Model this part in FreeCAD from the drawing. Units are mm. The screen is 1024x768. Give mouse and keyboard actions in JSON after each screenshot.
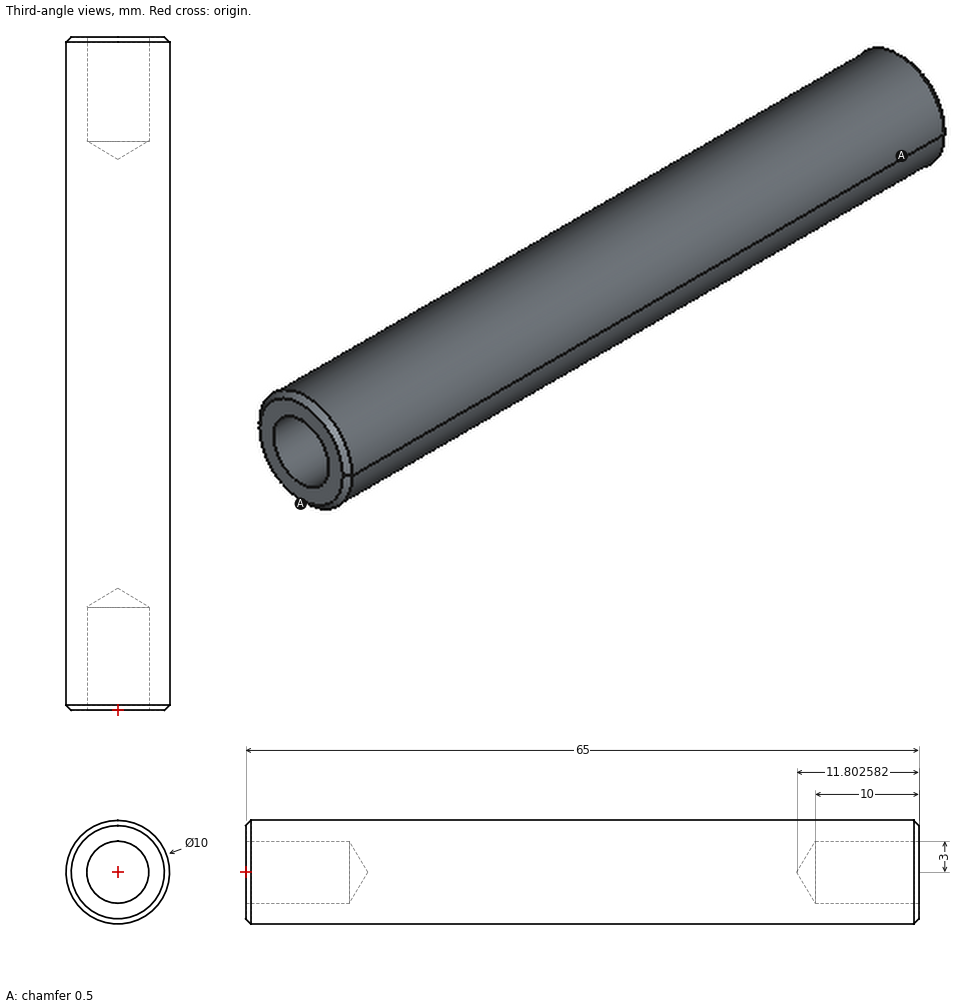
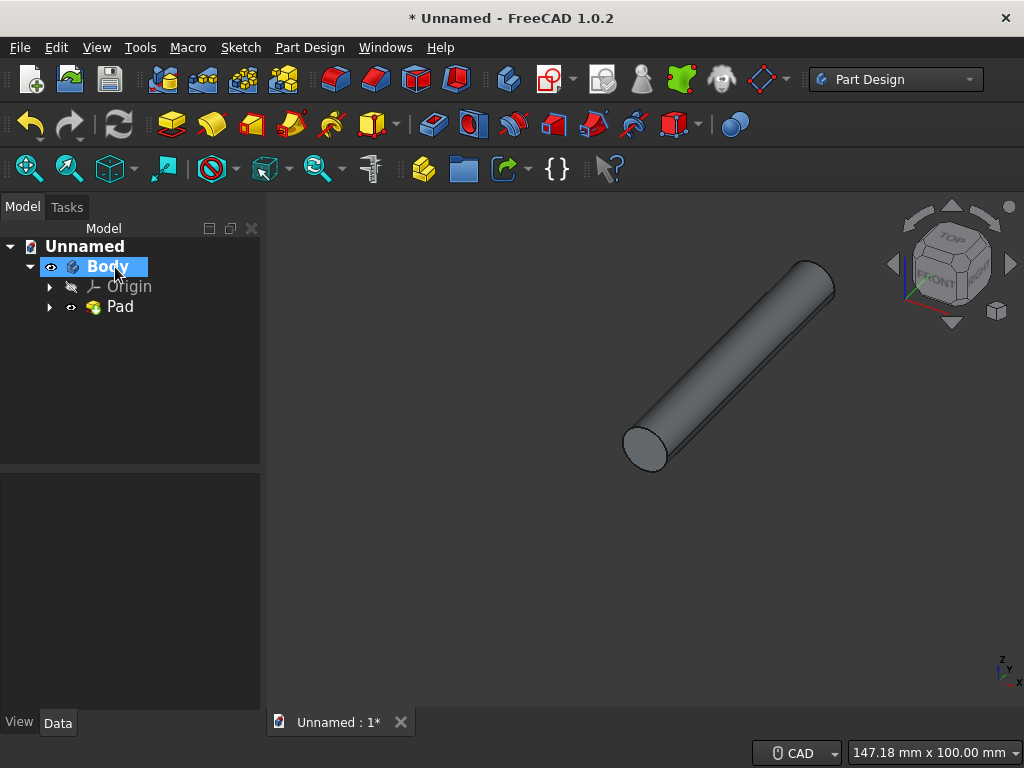
{"action": "left_click", "coordinate": [30, 170]}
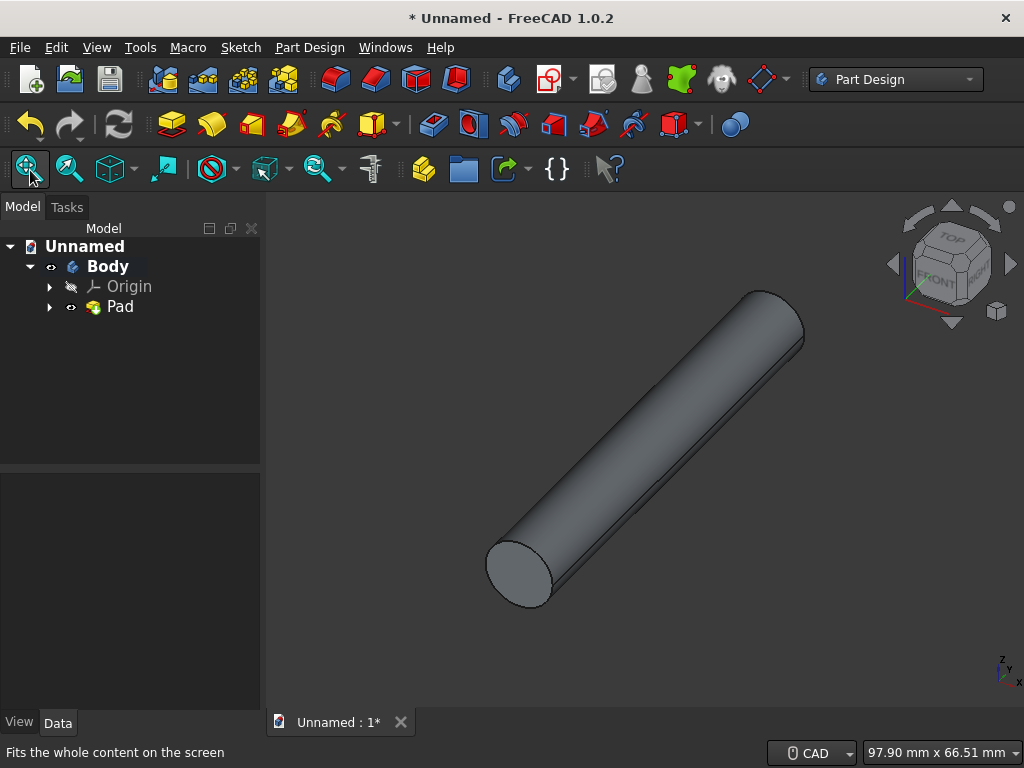
{"action": "left_click", "coordinate": [550, 80]}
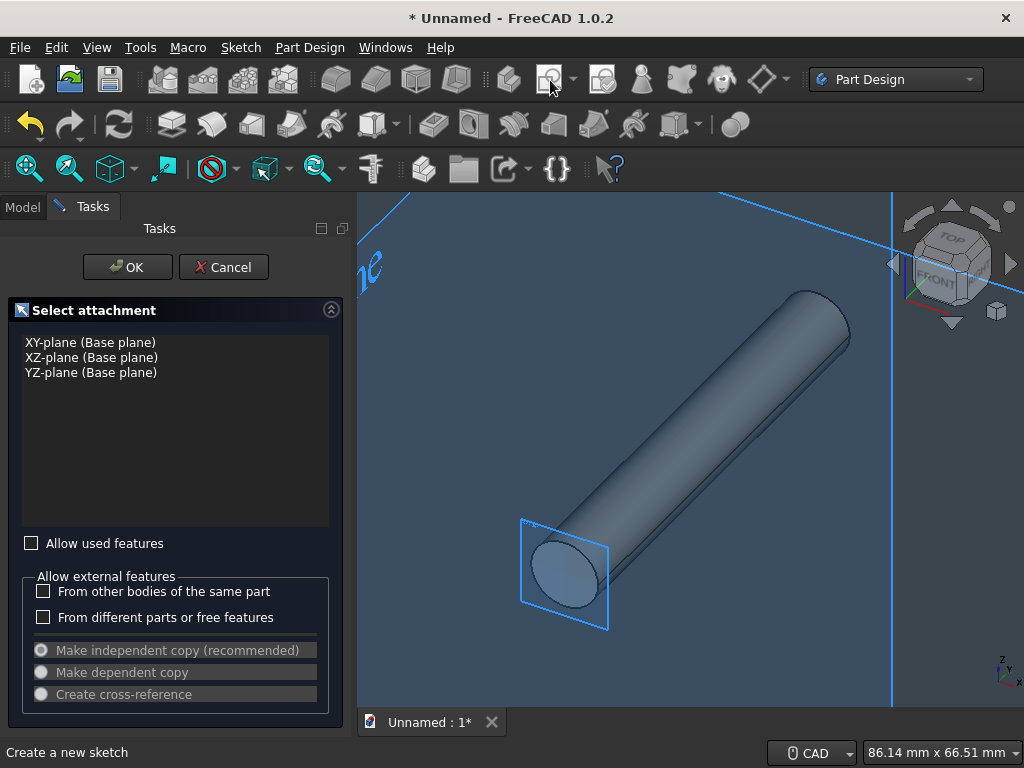
{"action": "left_click", "coordinate": [82, 372]}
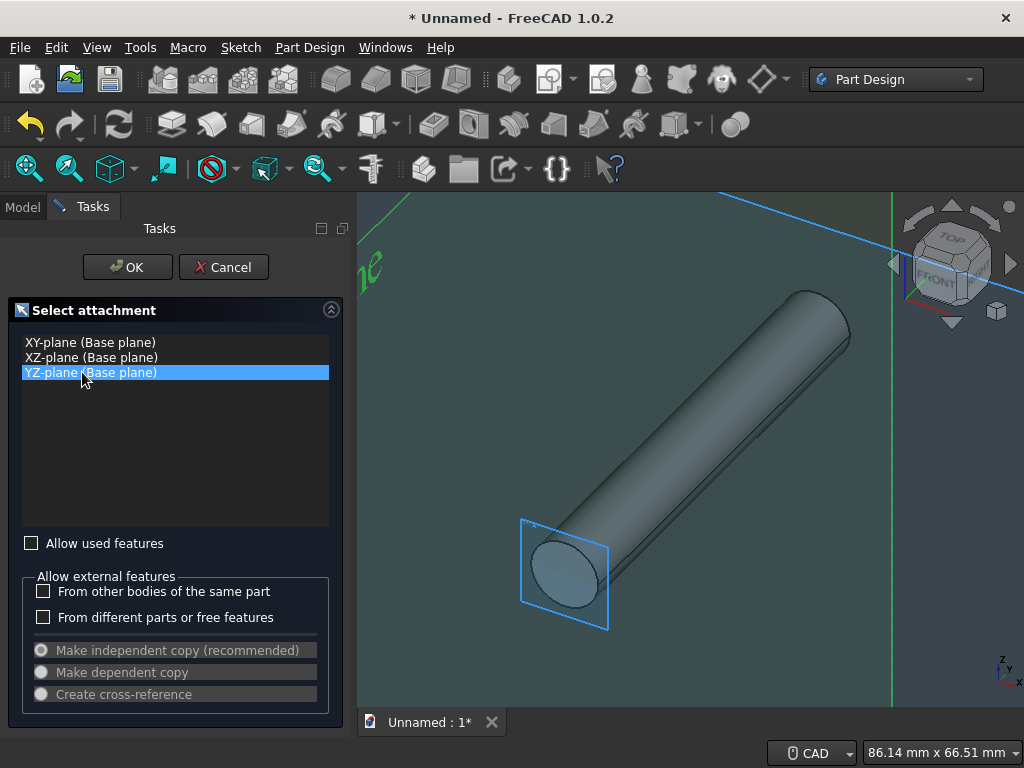
{"action": "left_click", "coordinate": [128, 267]}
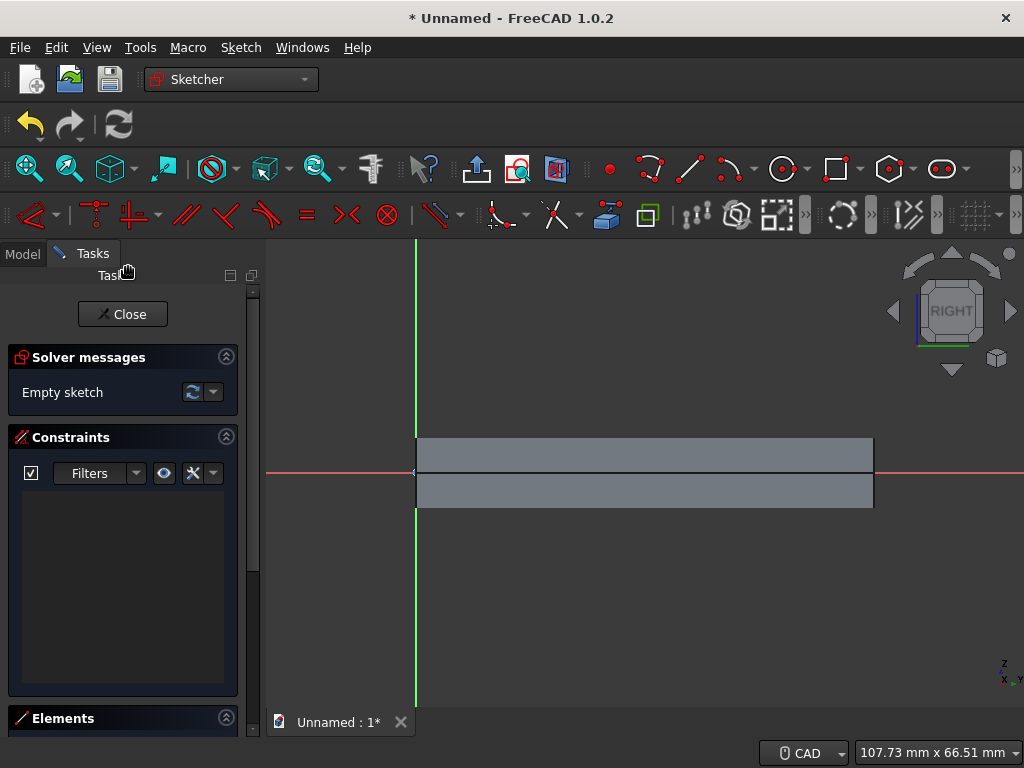
{"action": "left_click", "coordinate": [558, 170]}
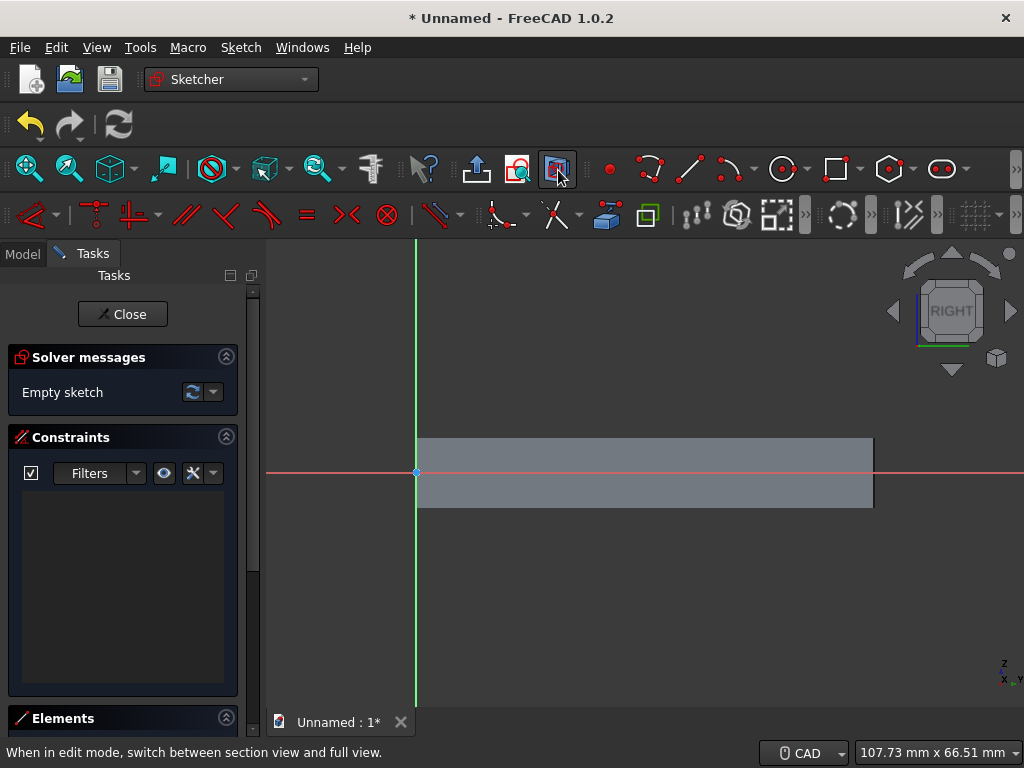
{"action": "scroll", "coordinate": [576, 473], "scroll_direction": "down", "scroll_amount": 5}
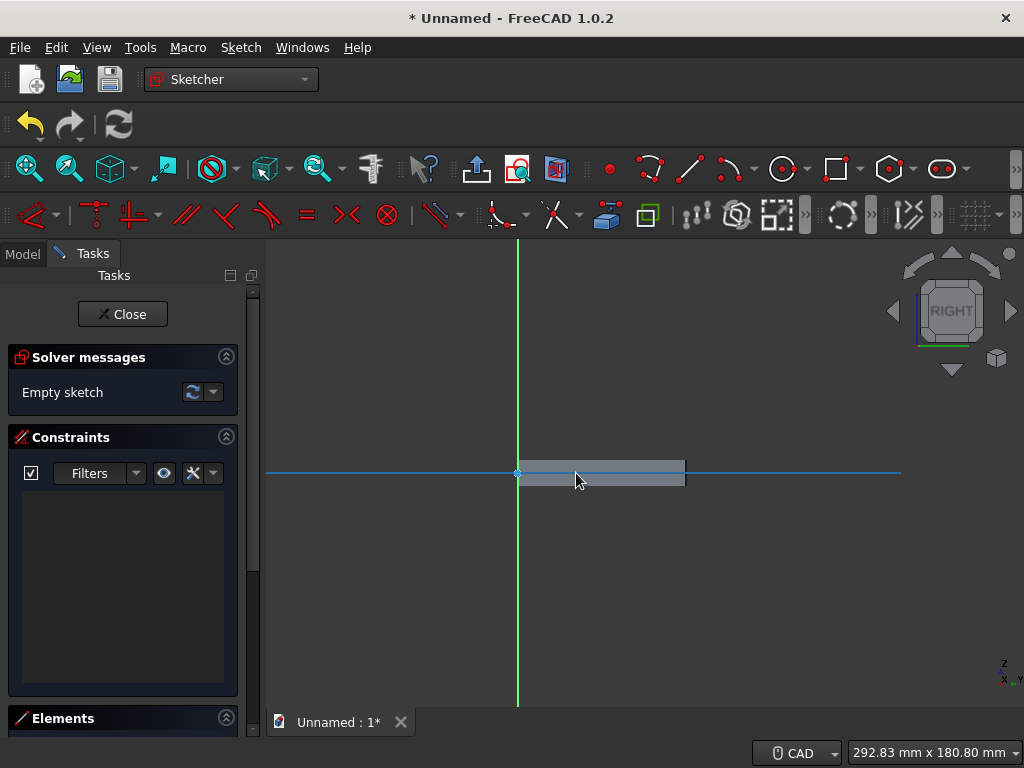
{"action": "scroll", "coordinate": [678, 469], "scroll_direction": "up", "scroll_amount": 13}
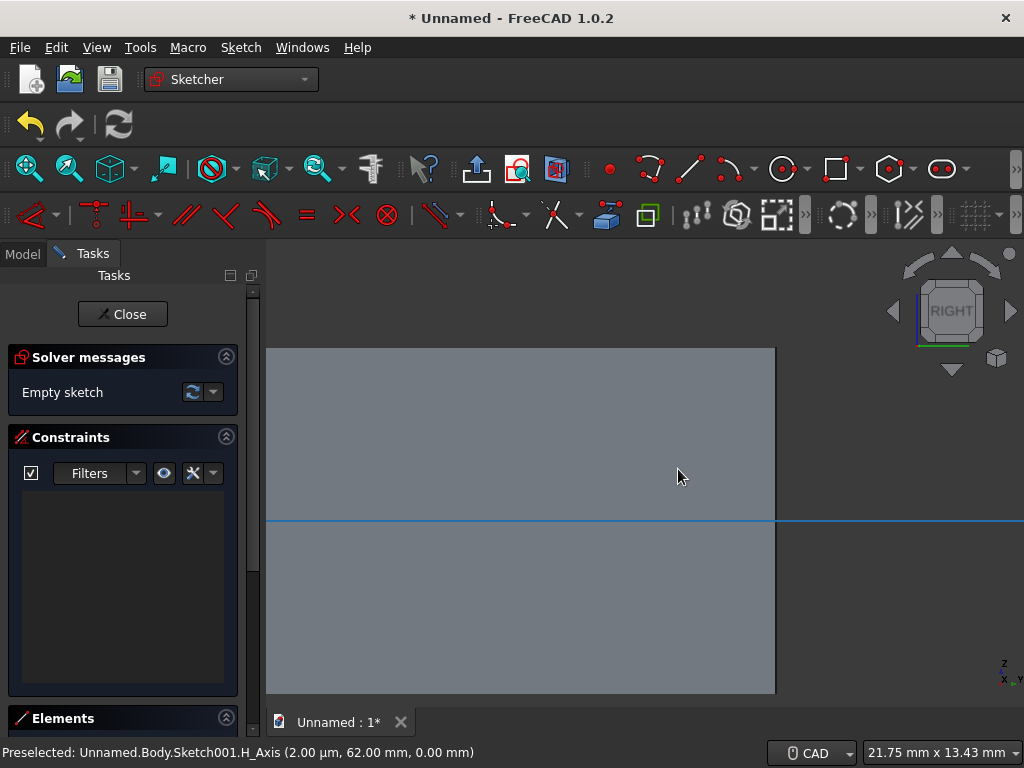
{"action": "left_click", "coordinate": [650, 170]}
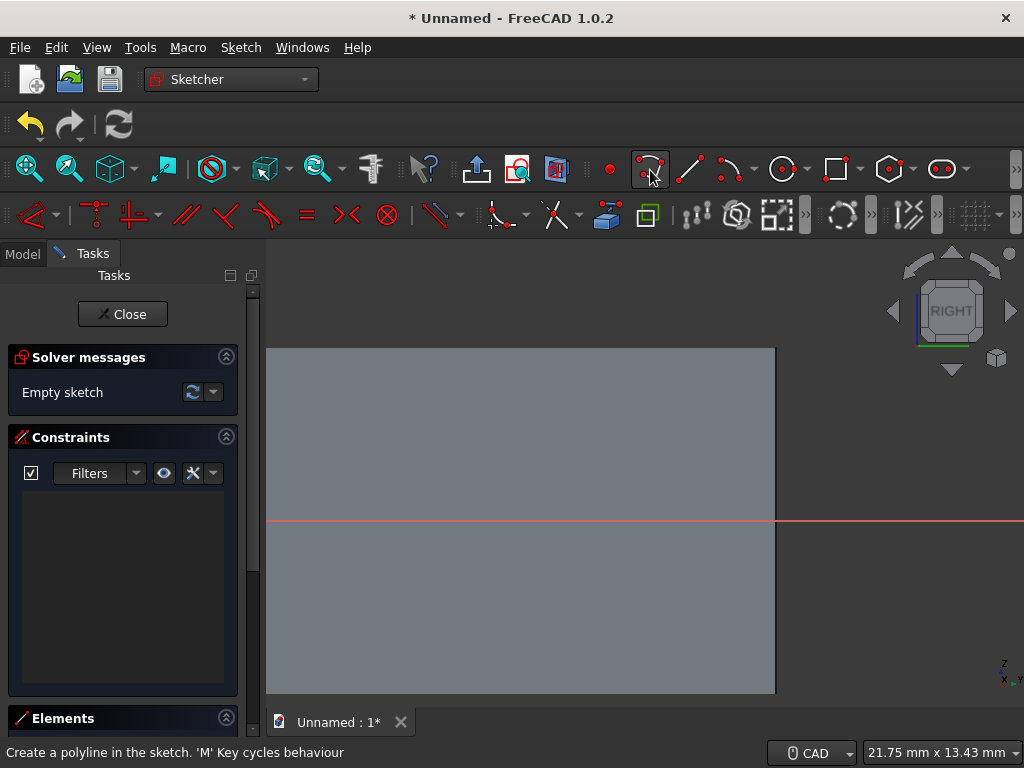
{"action": "left_click", "coordinate": [364, 521]}
{"action": "left_click", "coordinate": [776, 512]}
{"action": "left_click", "coordinate": [776, 416]}
{"action": "left_click", "coordinate": [427, 416]}
{"action": "left_click", "coordinate": [364, 521]}
{"action": "key", "text": "Escape"}
{"action": "key", "text": "Escape"}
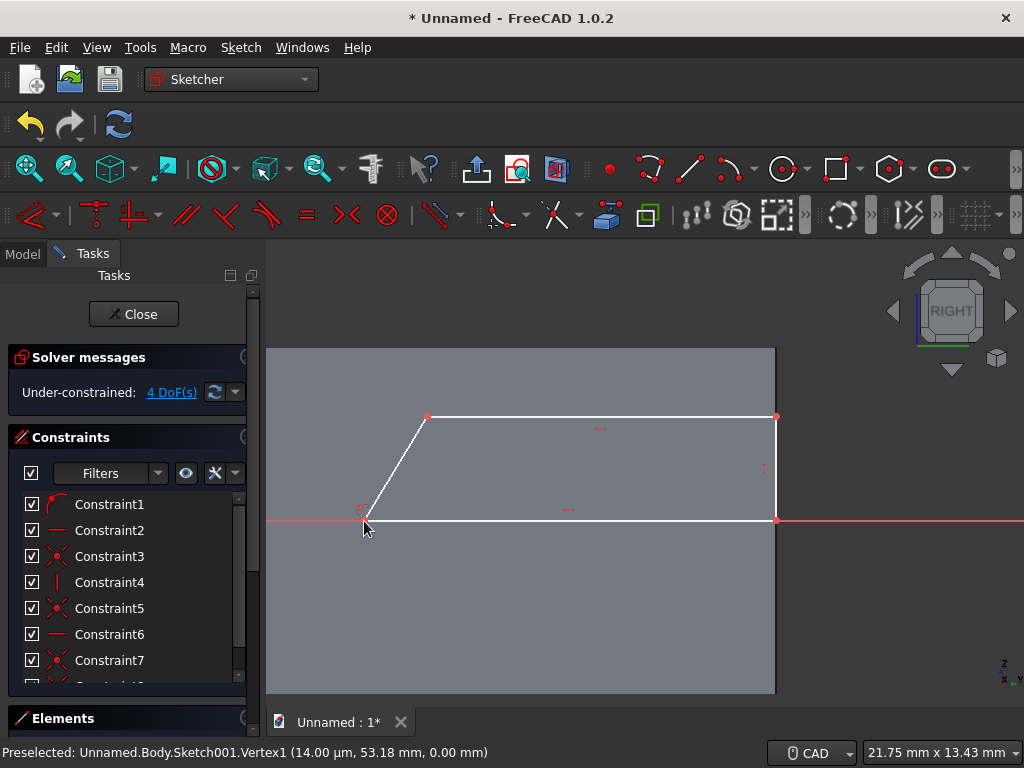
{"action": "left_click", "coordinate": [32, 216]}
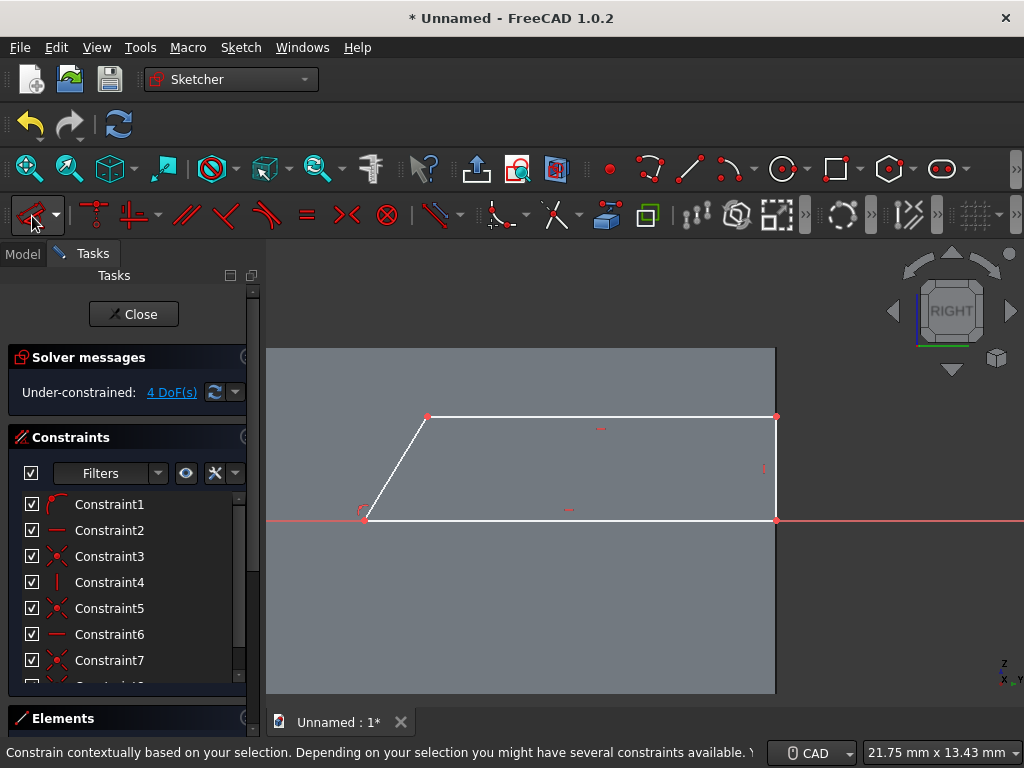
{"action": "left_click", "coordinate": [776, 490]}
{"action": "left_click", "coordinate": [810, 469]}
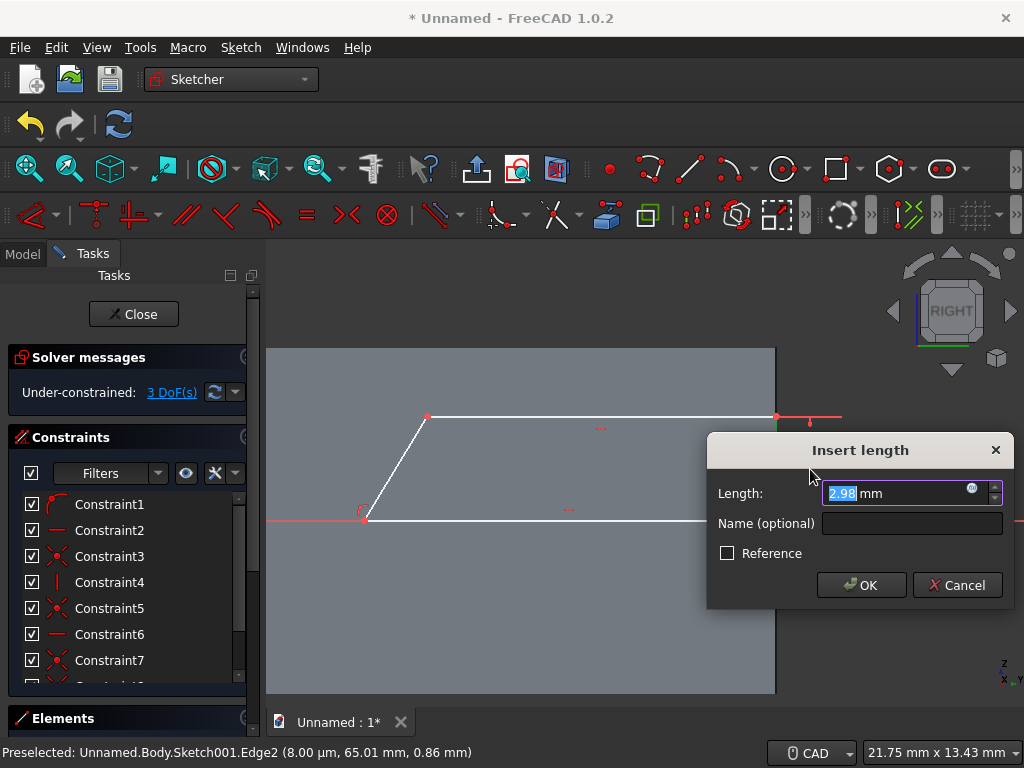
{"action": "type", "text": "3"}
{"action": "key", "text": "Return"}